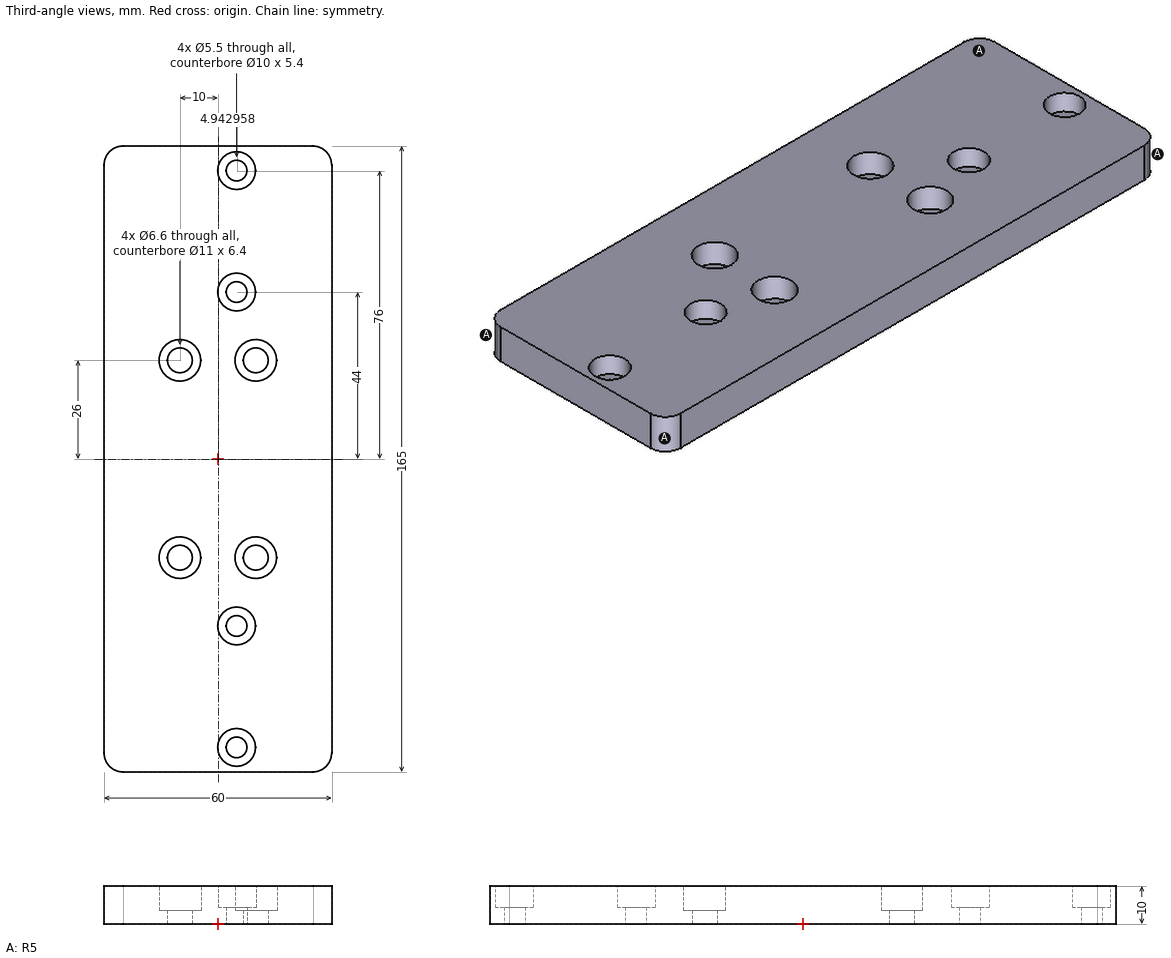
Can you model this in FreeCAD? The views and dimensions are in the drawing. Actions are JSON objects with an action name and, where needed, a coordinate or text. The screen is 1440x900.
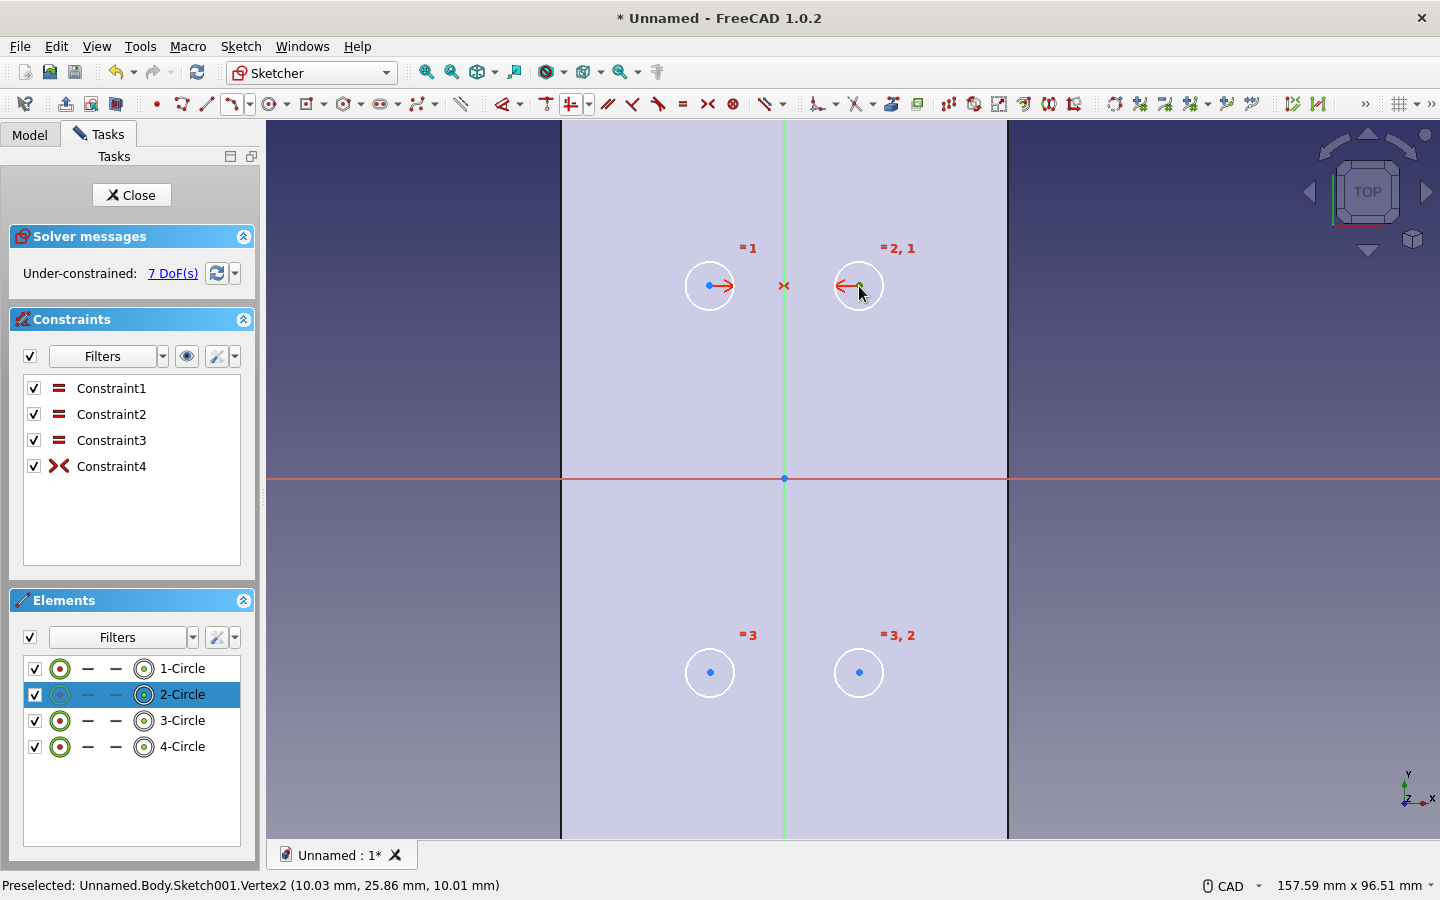
{"action": "left_click", "coordinate": [859, 673]}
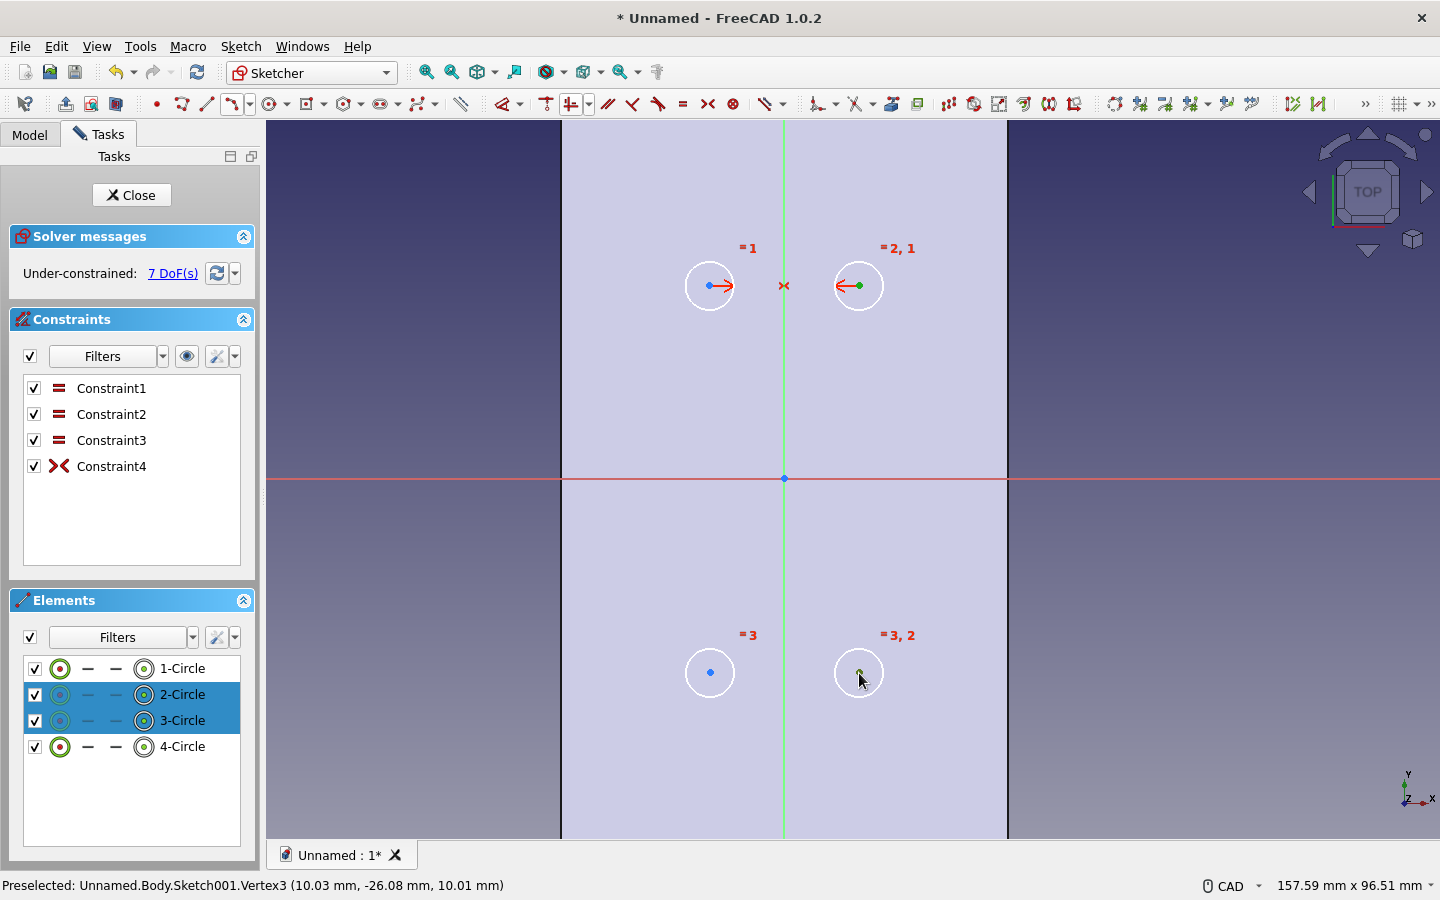
{"action": "left_click", "coordinate": [364, 479]}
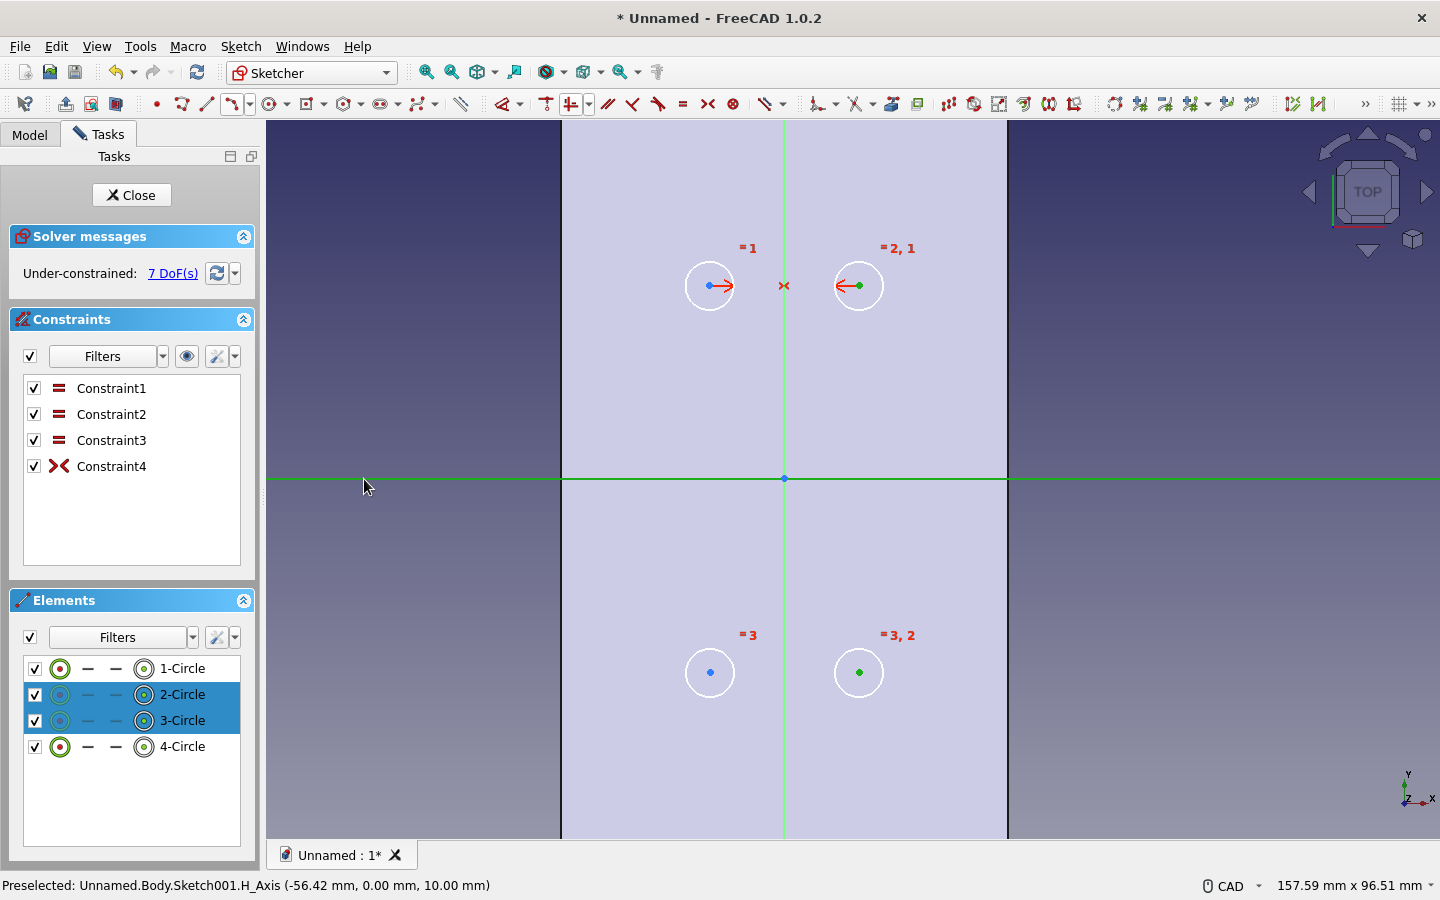
{"action": "left_click", "coordinate": [708, 104]}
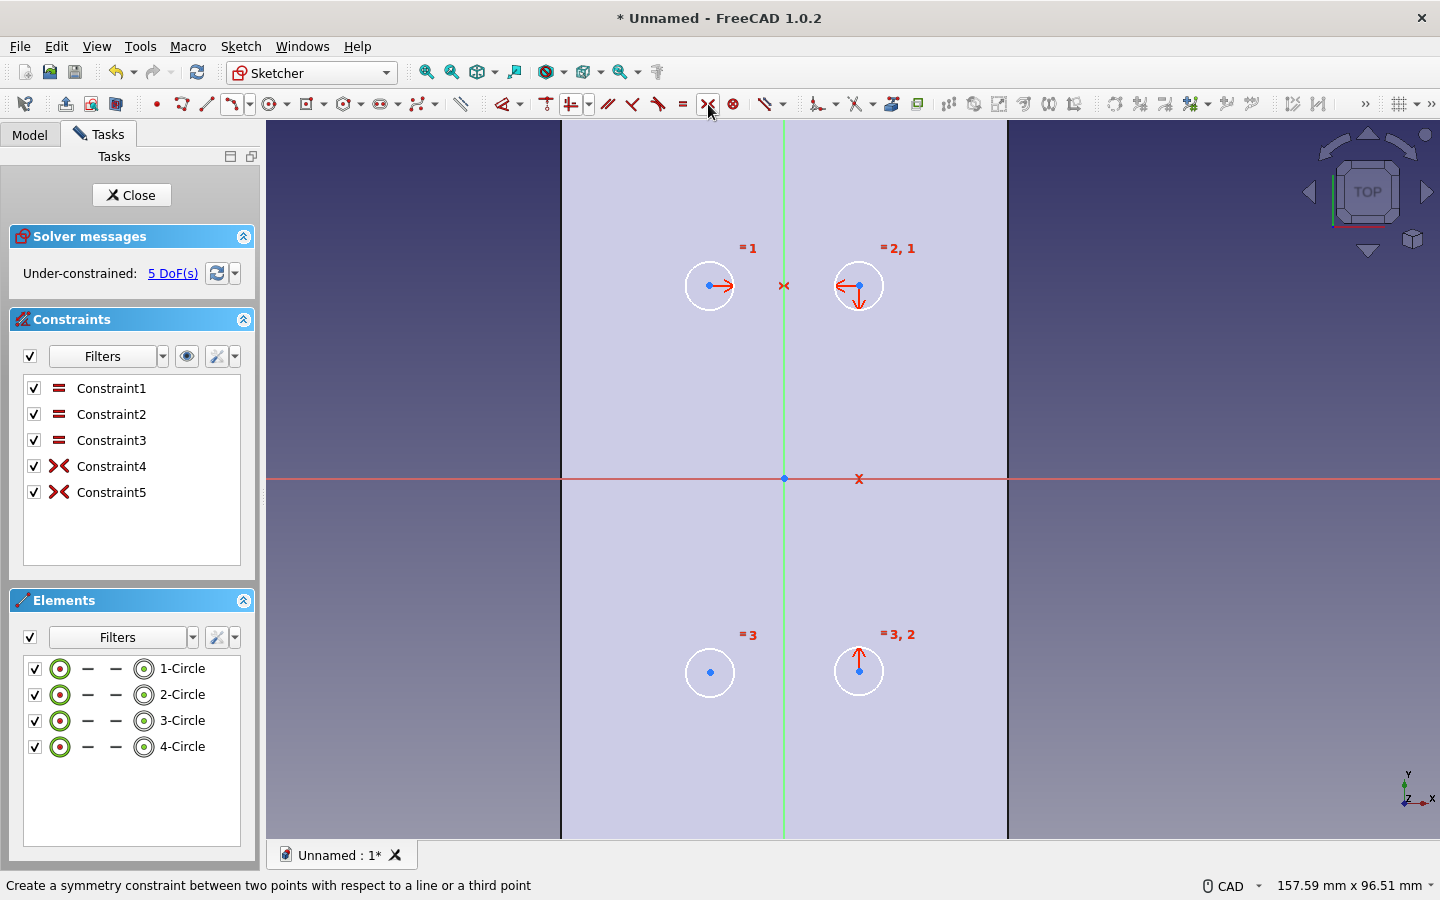
{"action": "left_click", "coordinate": [710, 286]}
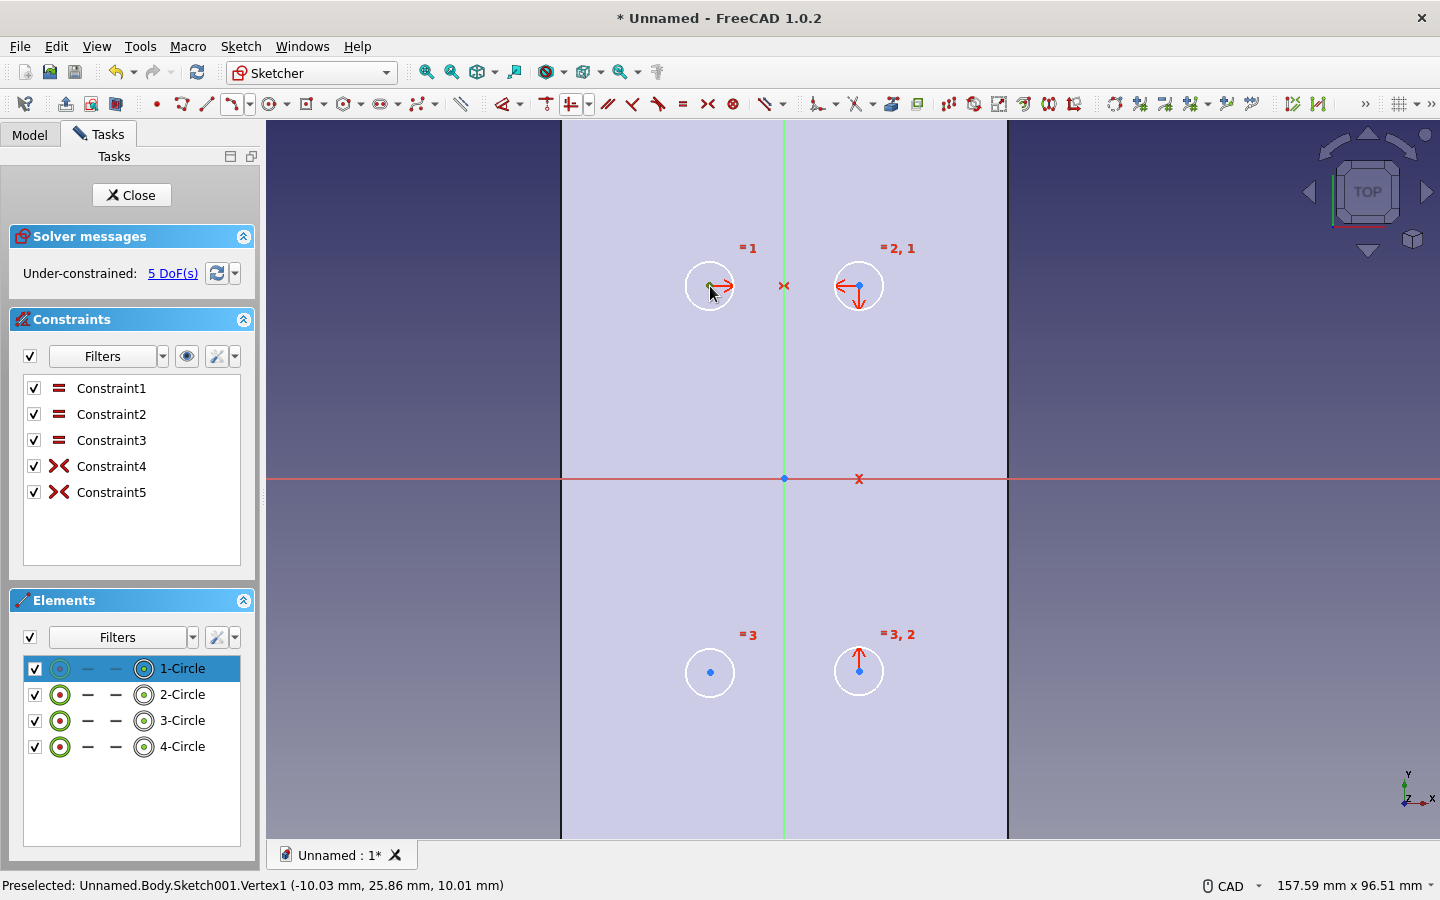
{"action": "left_click", "coordinate": [710, 673]}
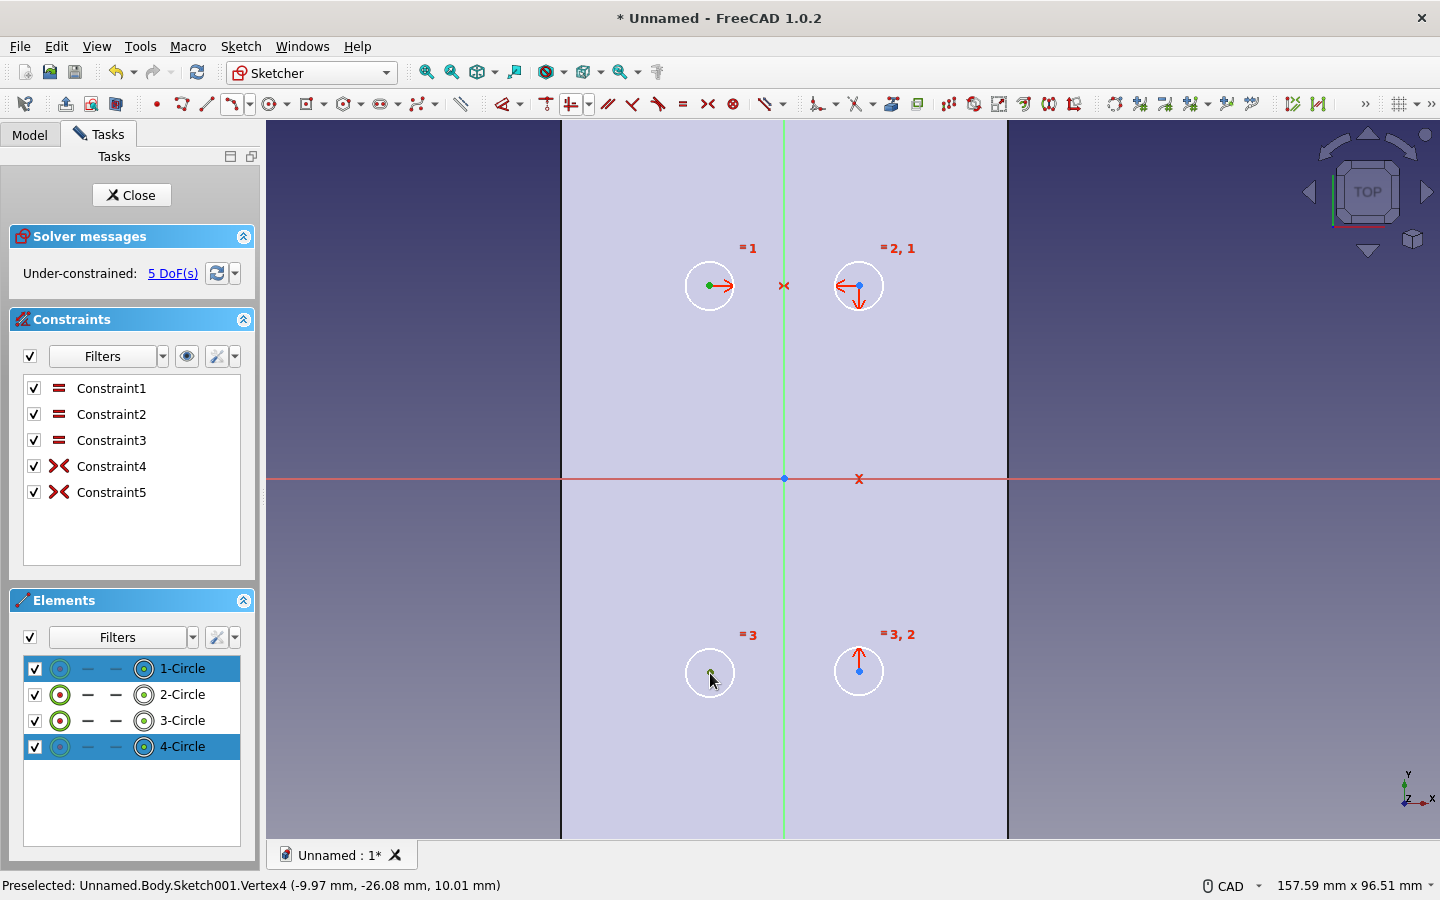
{"action": "left_click", "coordinate": [364, 479]}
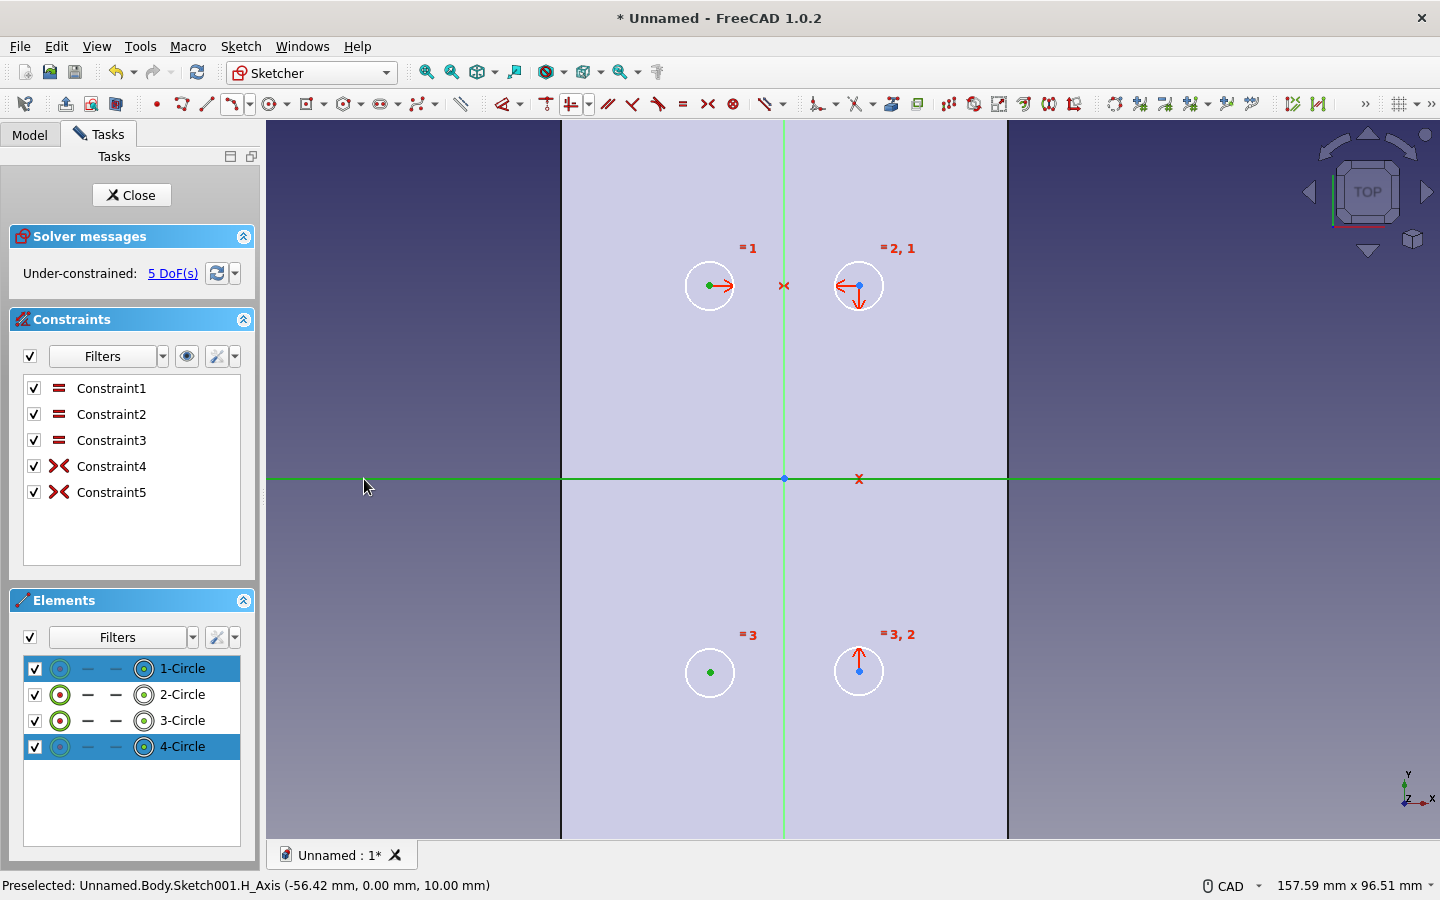
{"action": "key", "text": "s"}